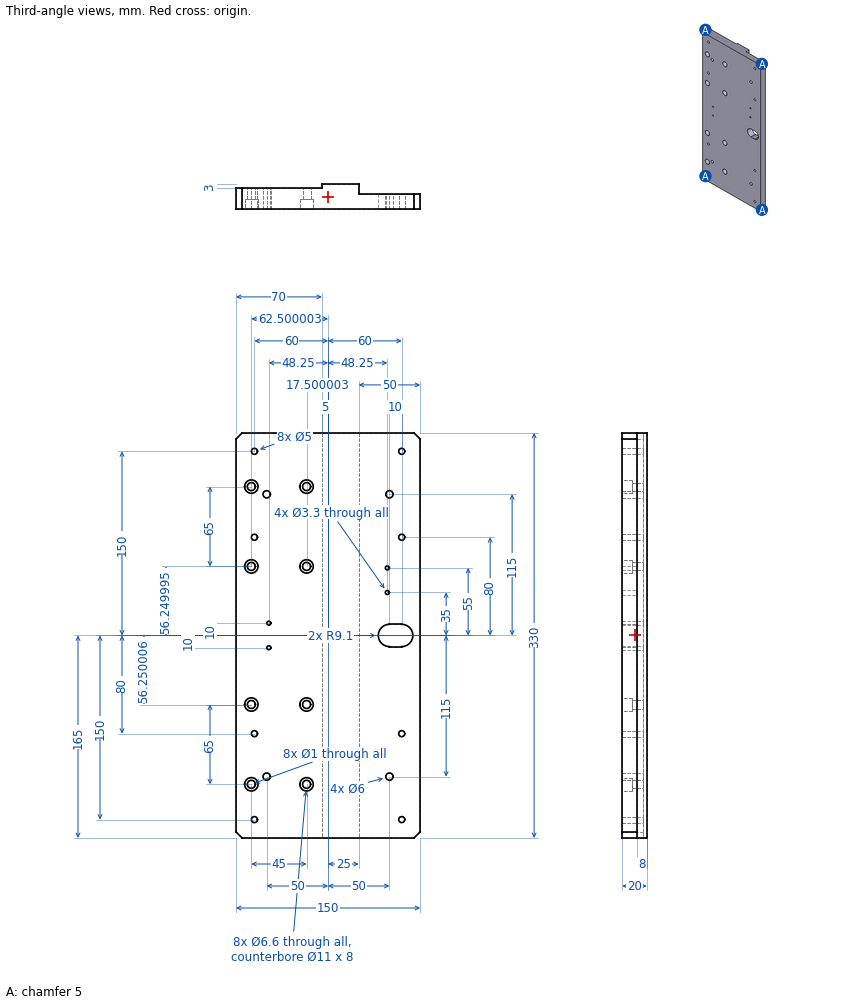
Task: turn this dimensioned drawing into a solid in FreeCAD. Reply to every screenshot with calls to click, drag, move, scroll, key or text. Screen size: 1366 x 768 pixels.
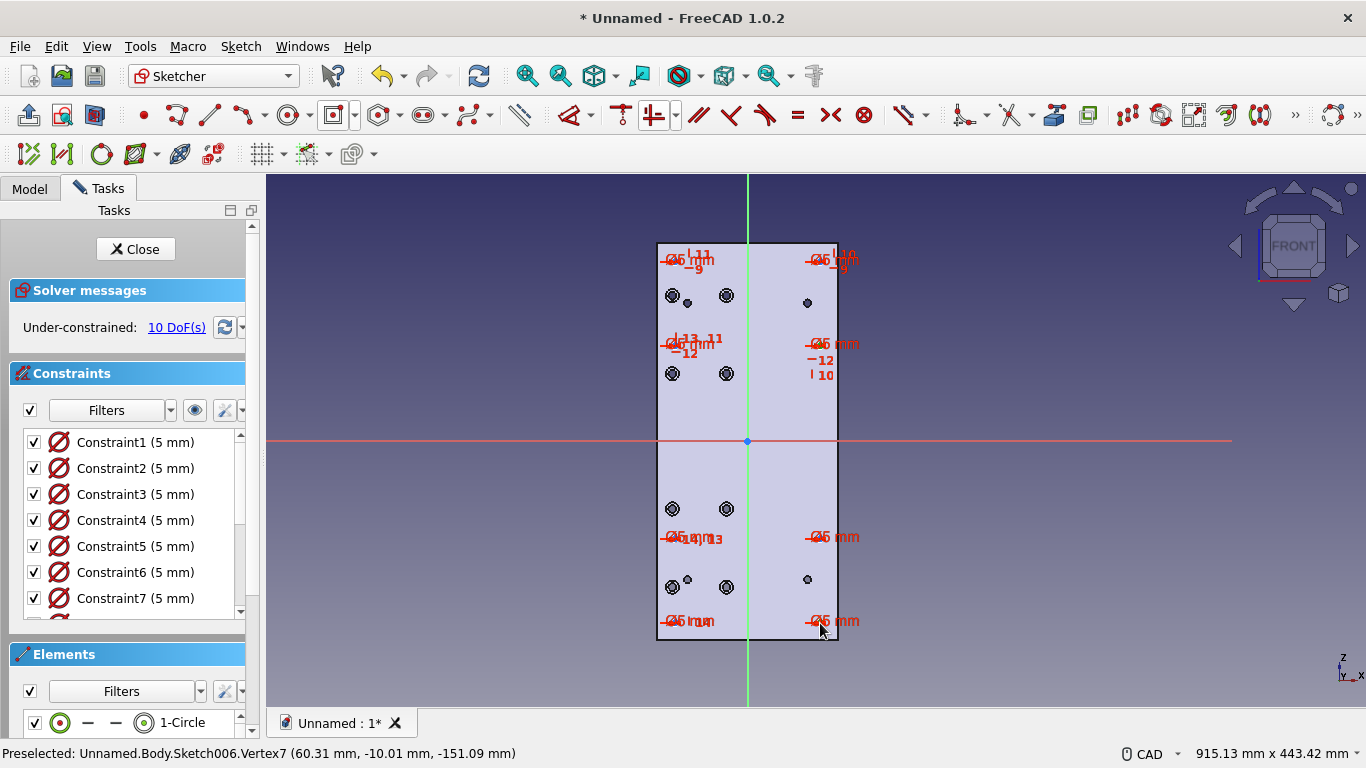
key(v)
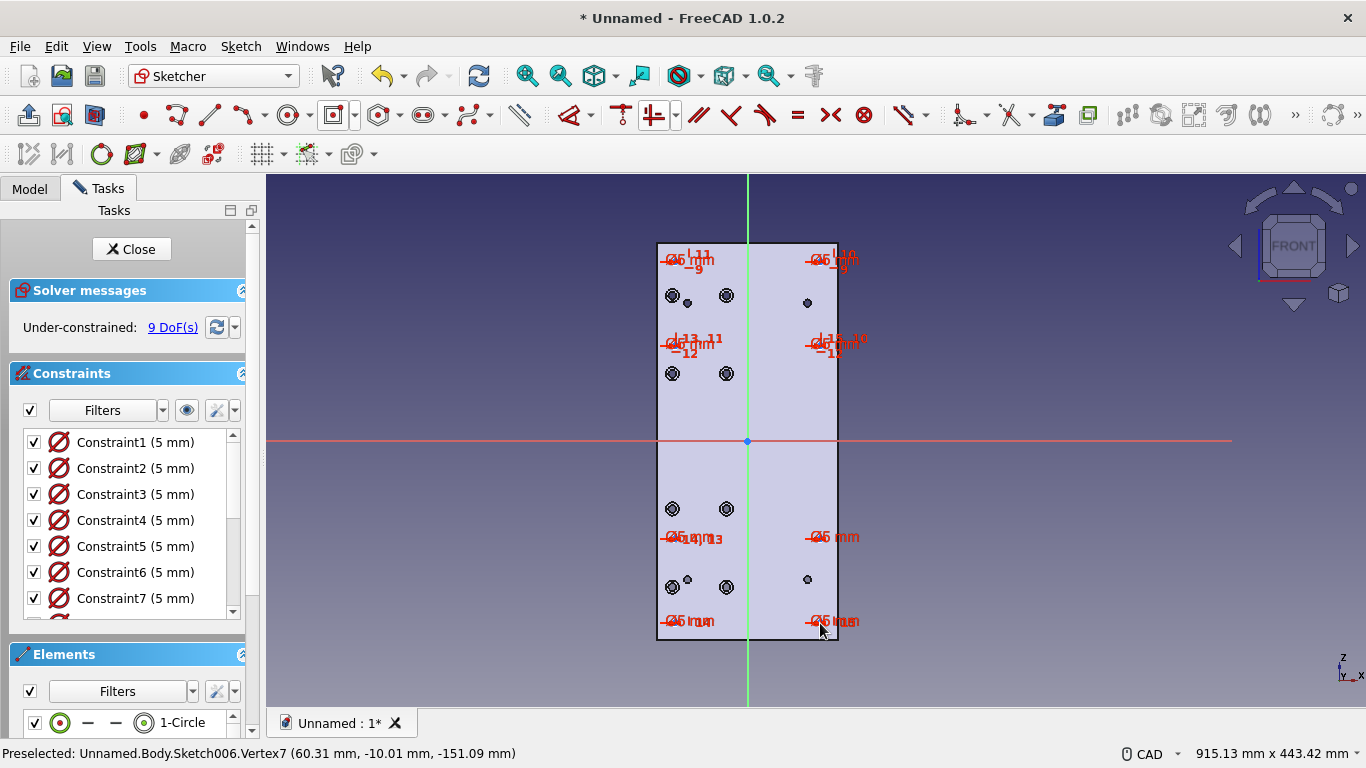
click(675, 623)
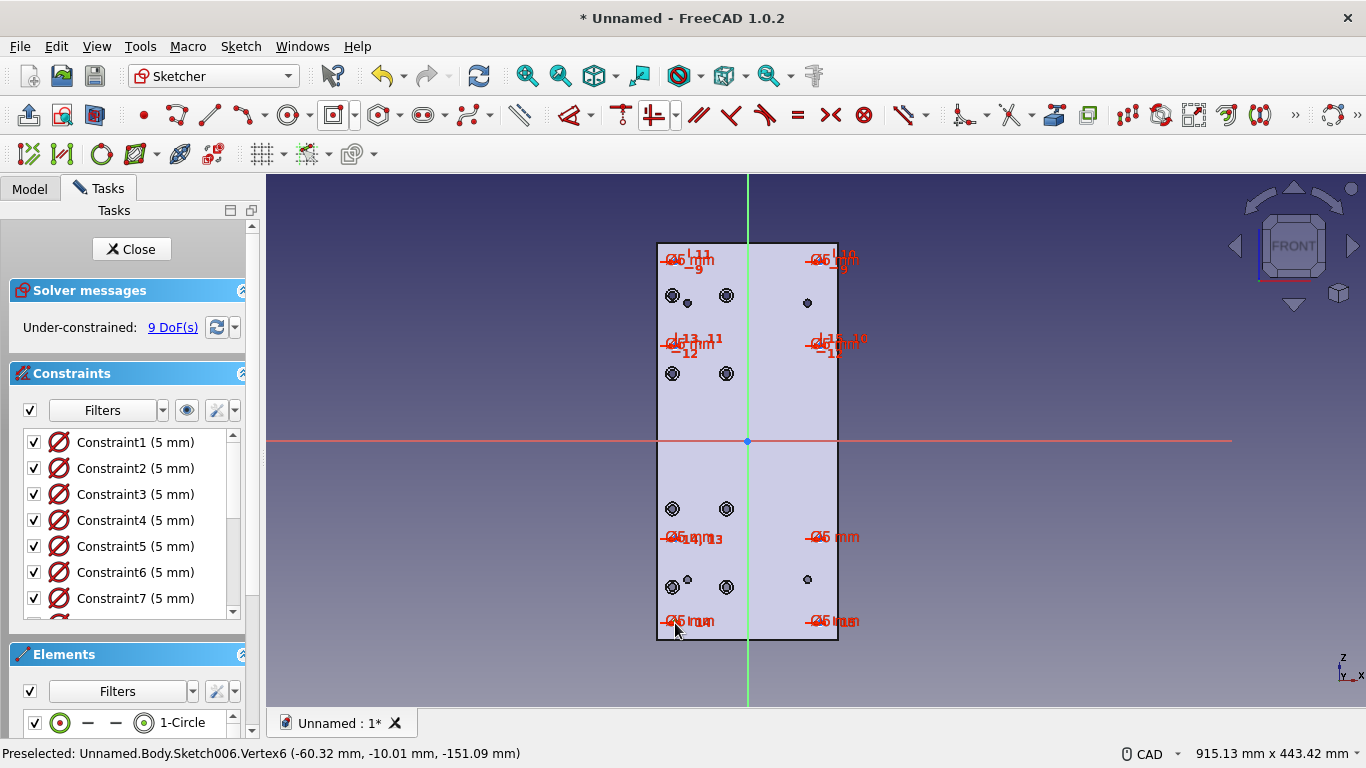
click(820, 623)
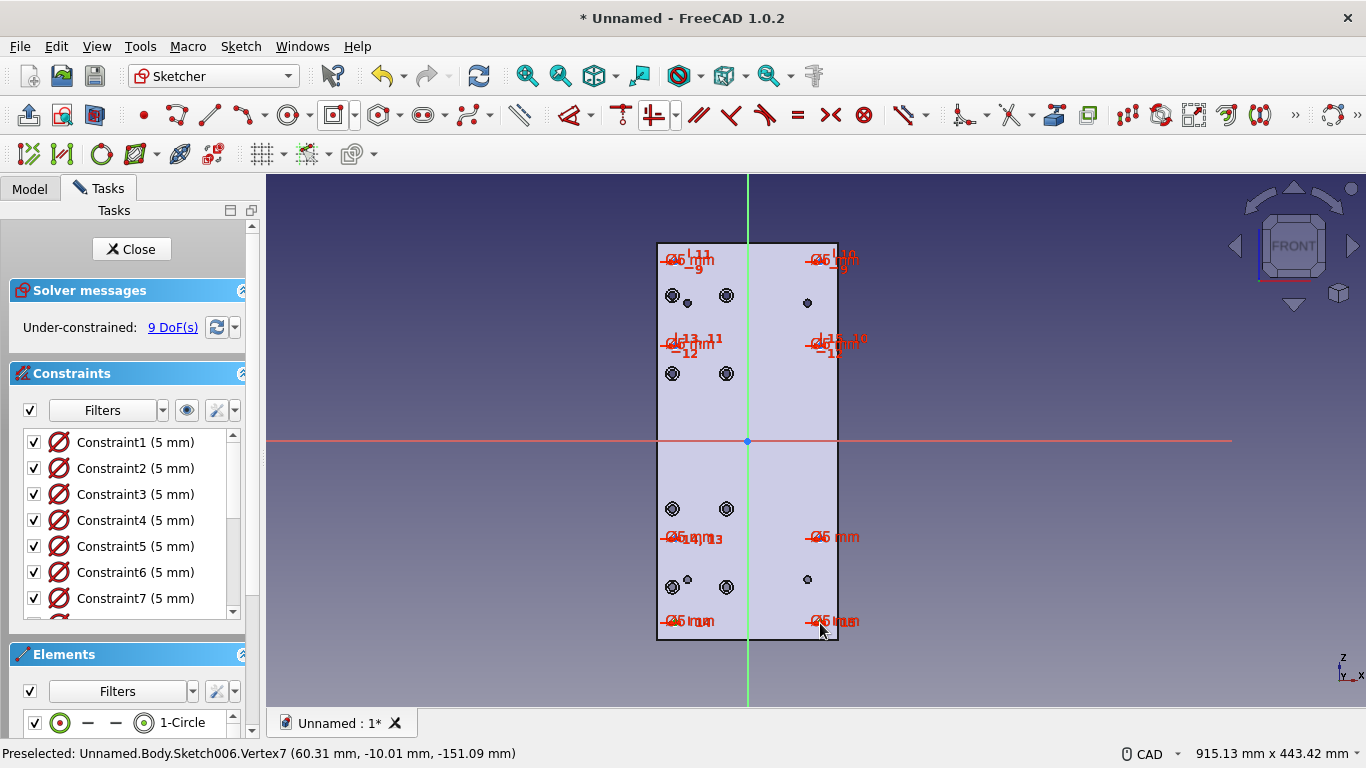
key(h)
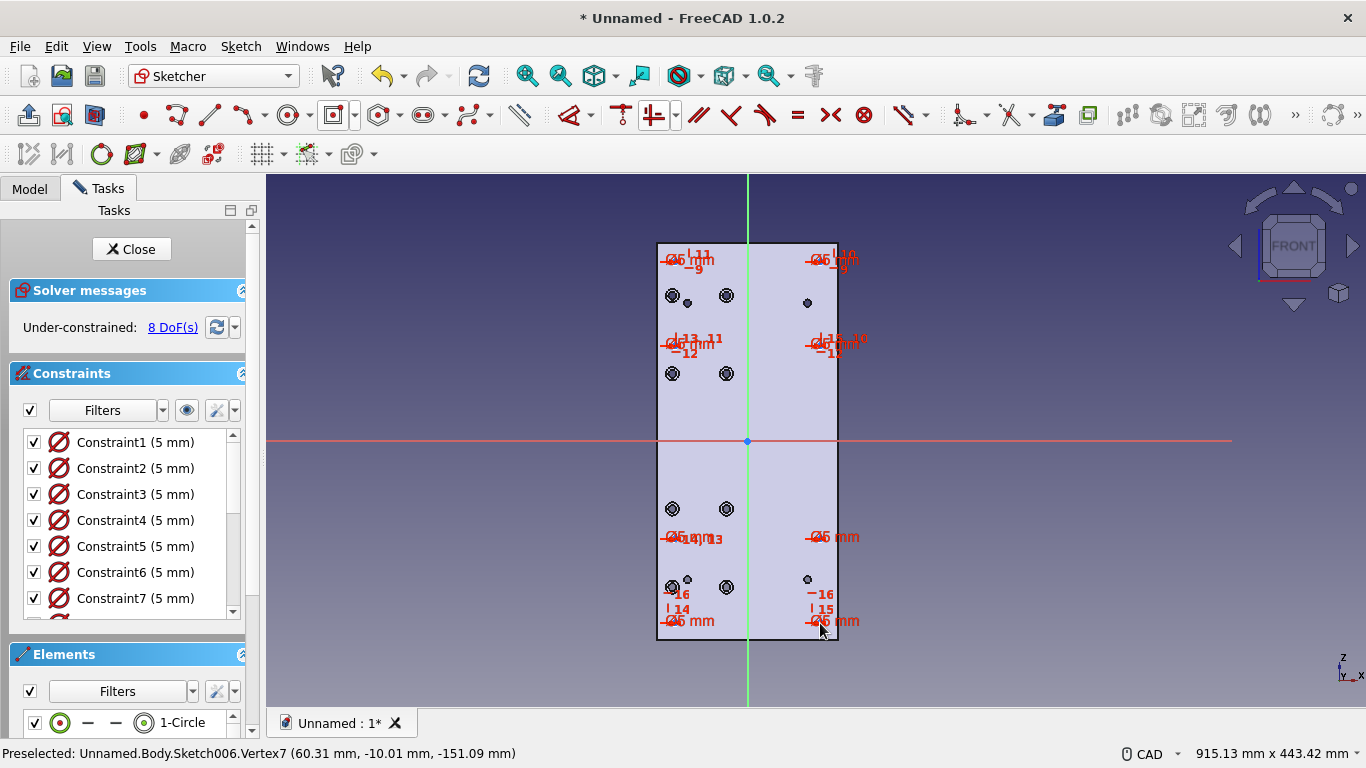
click(820, 623)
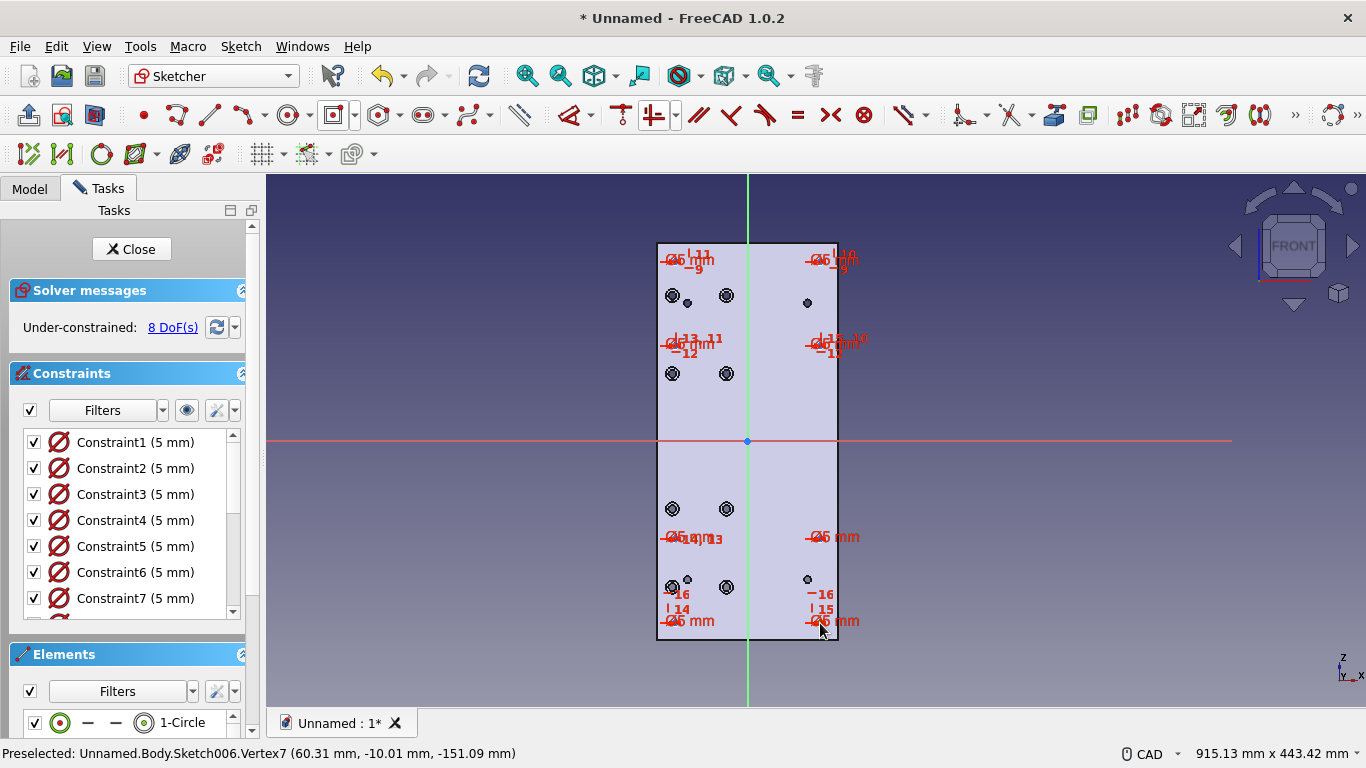
click(820, 539)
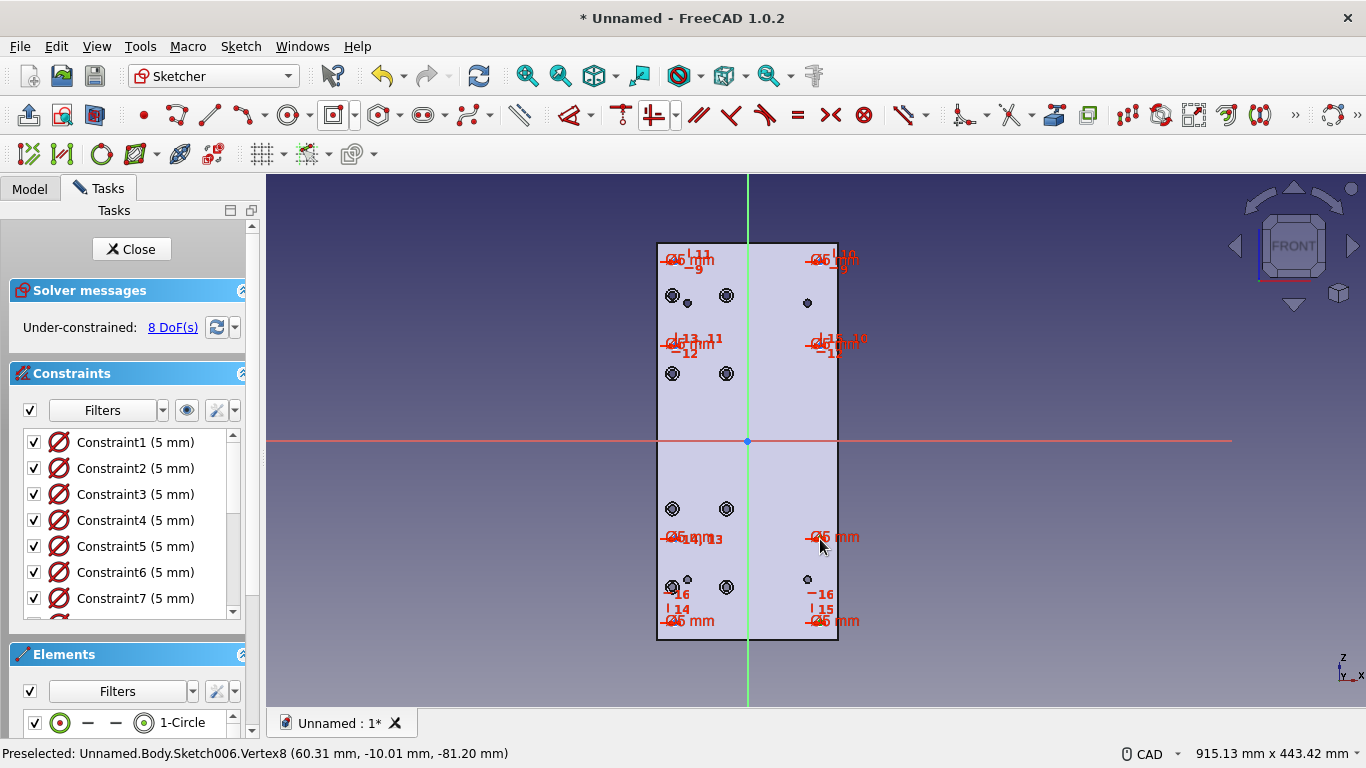
key(v)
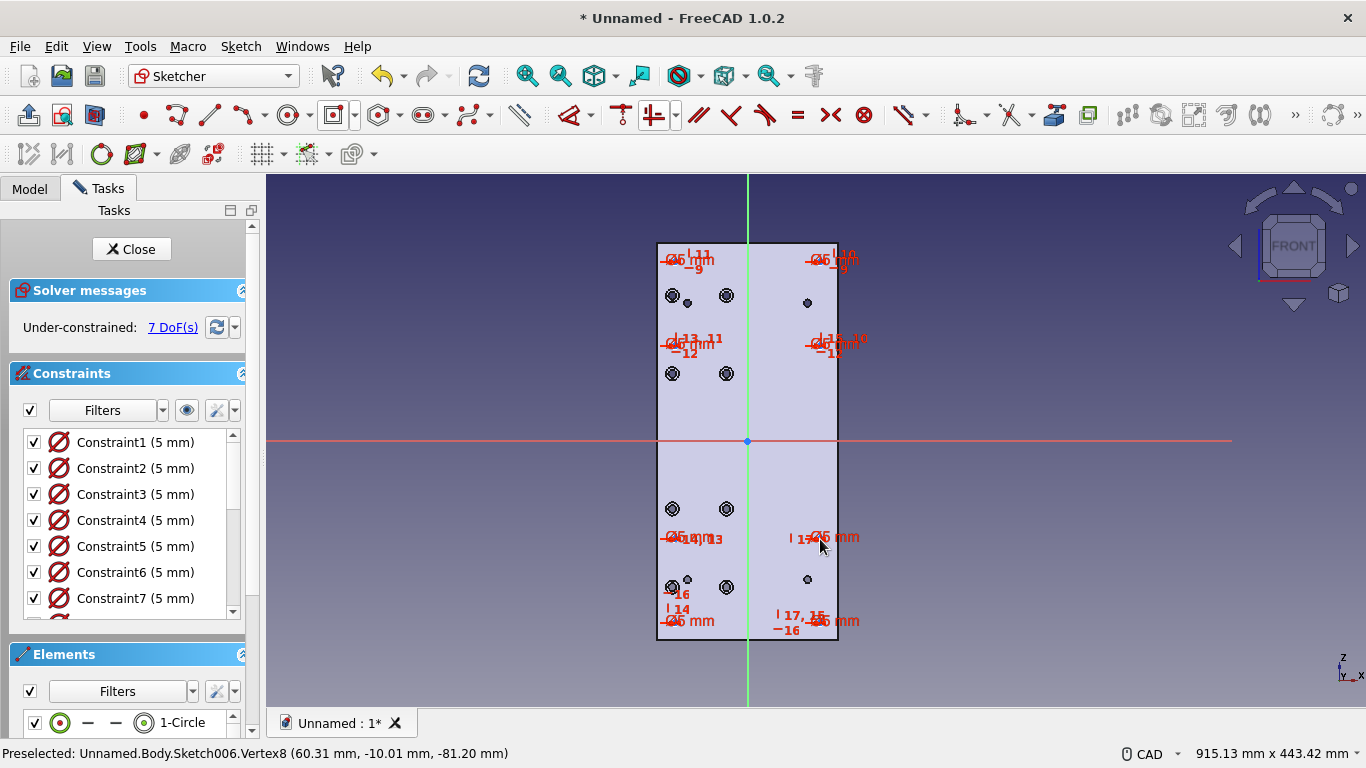
click(675, 539)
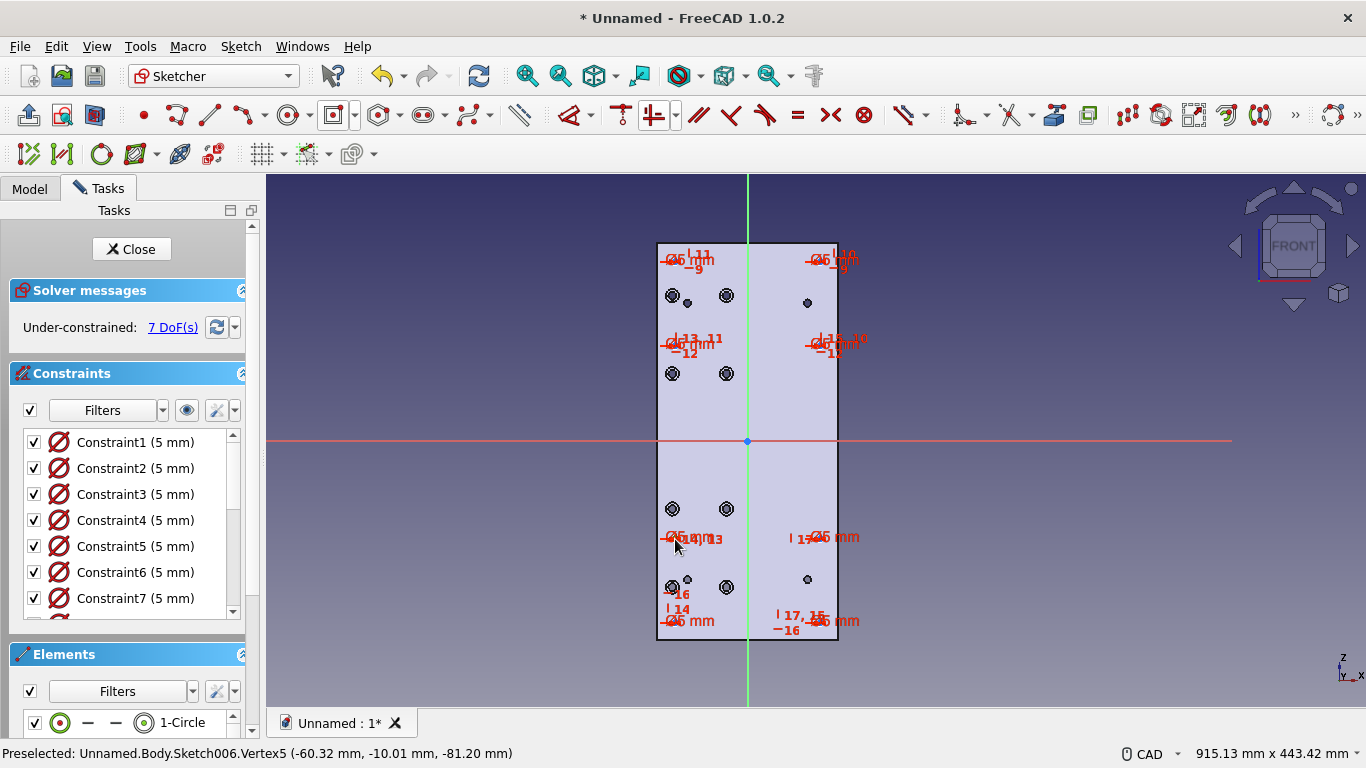
click(820, 539)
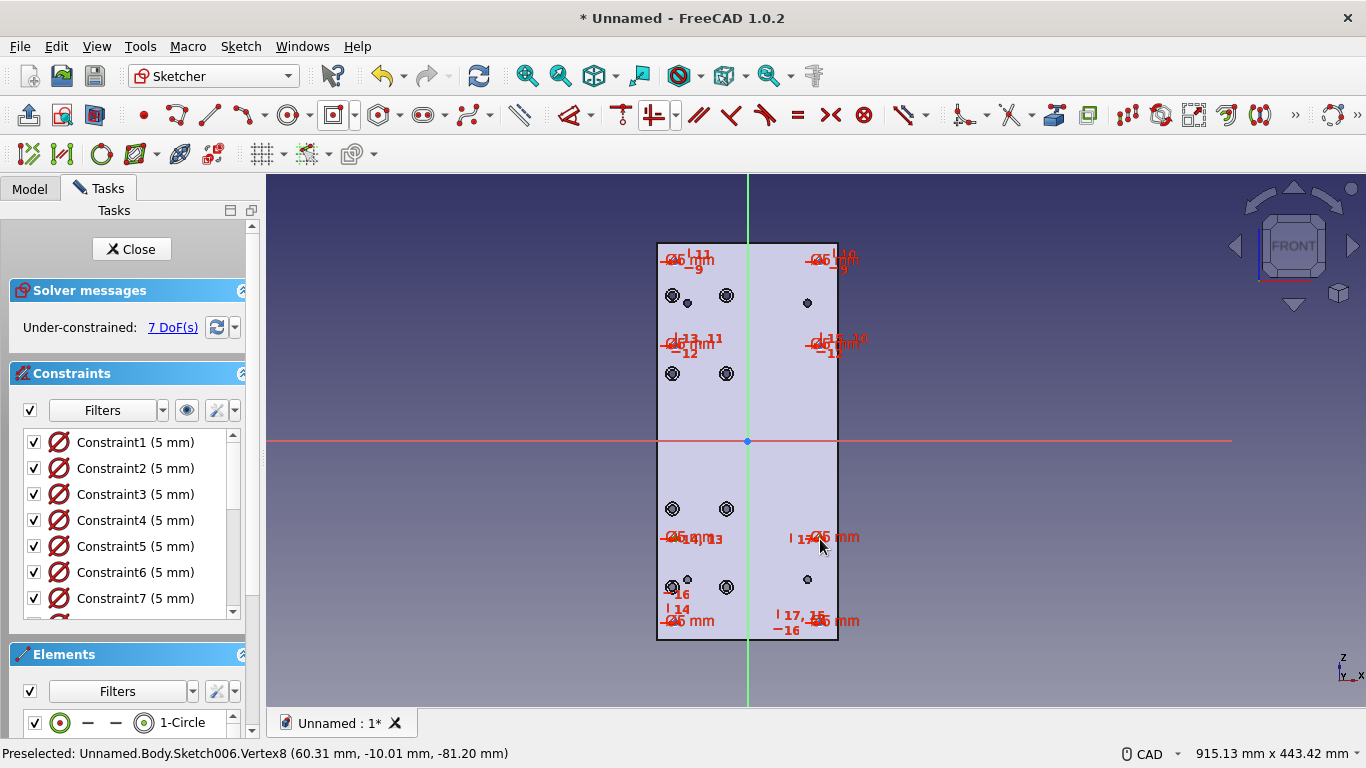
click(676, 116)